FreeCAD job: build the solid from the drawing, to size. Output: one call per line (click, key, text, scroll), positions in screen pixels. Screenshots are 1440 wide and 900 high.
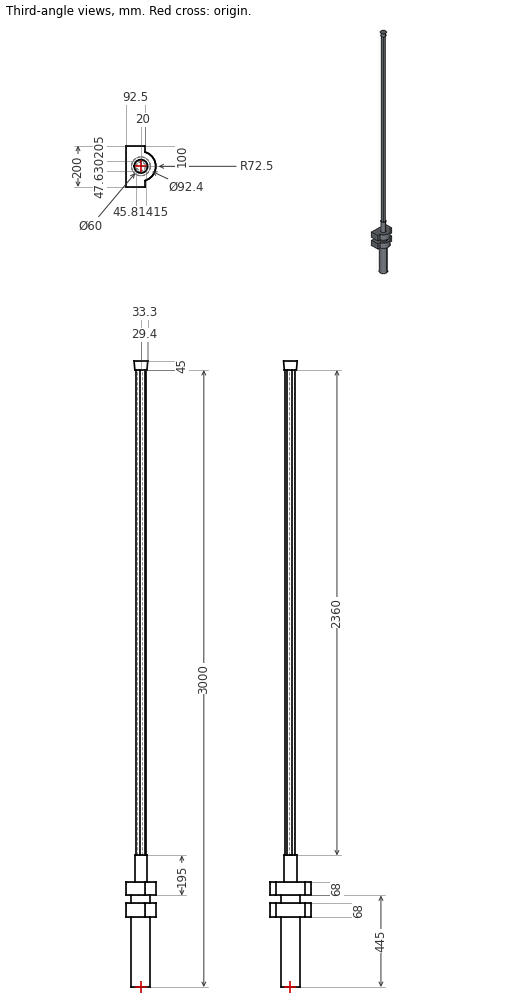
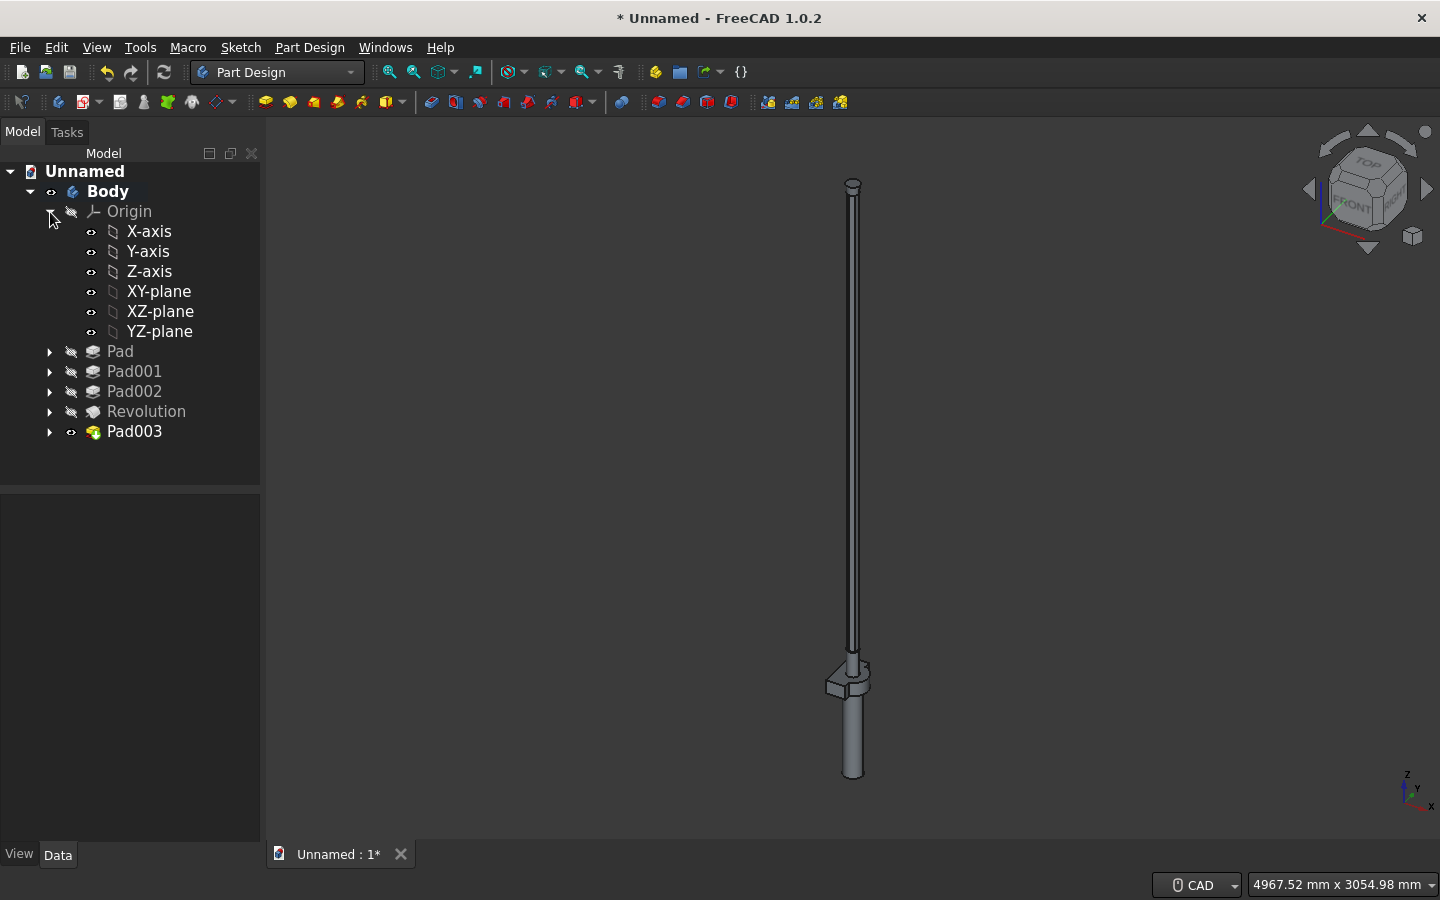
click(136, 292)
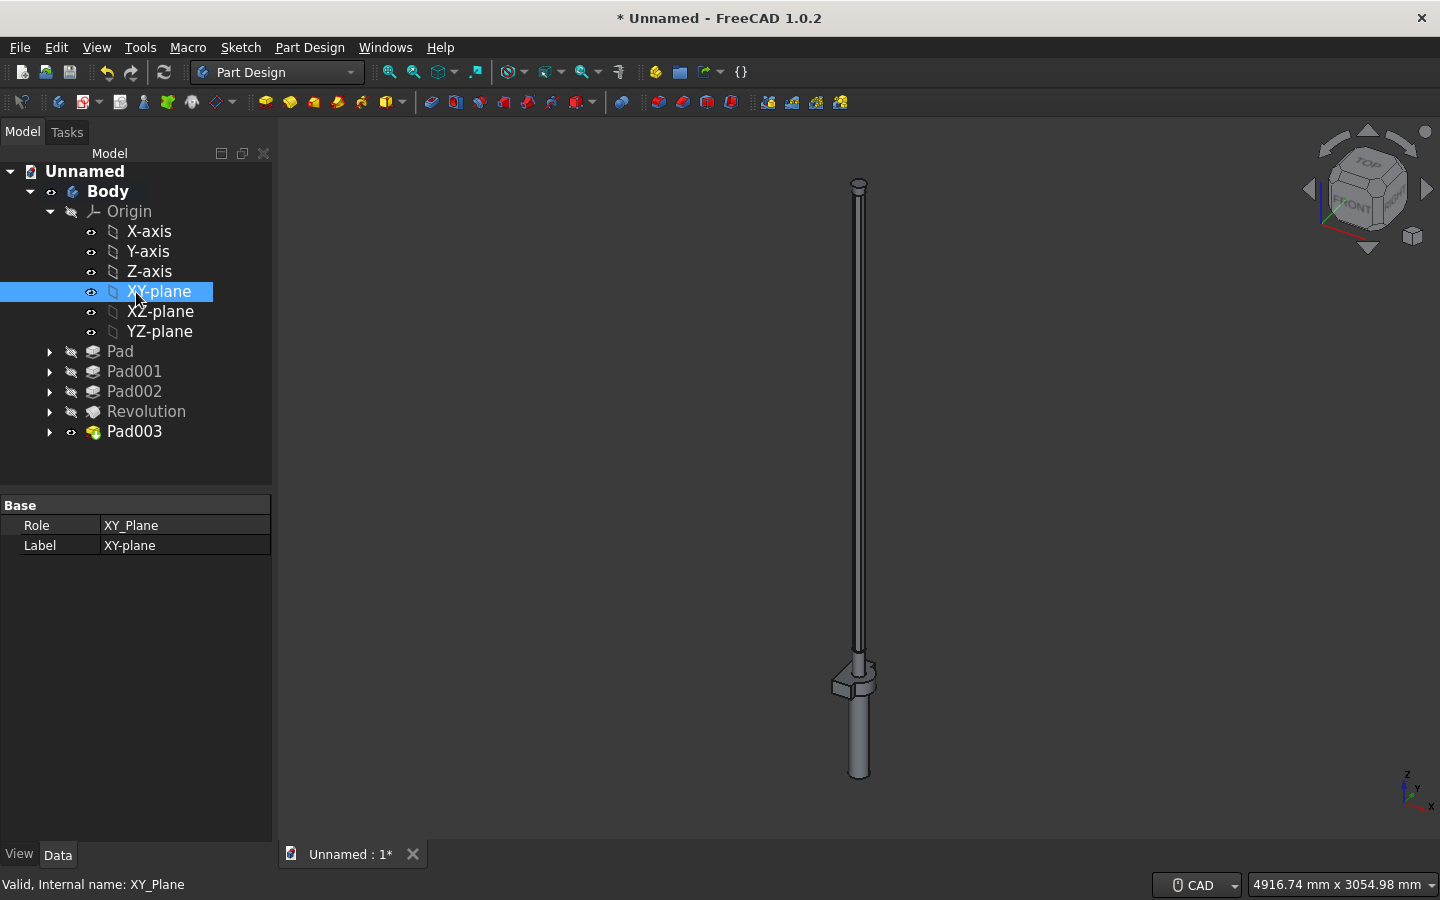
click(216, 102)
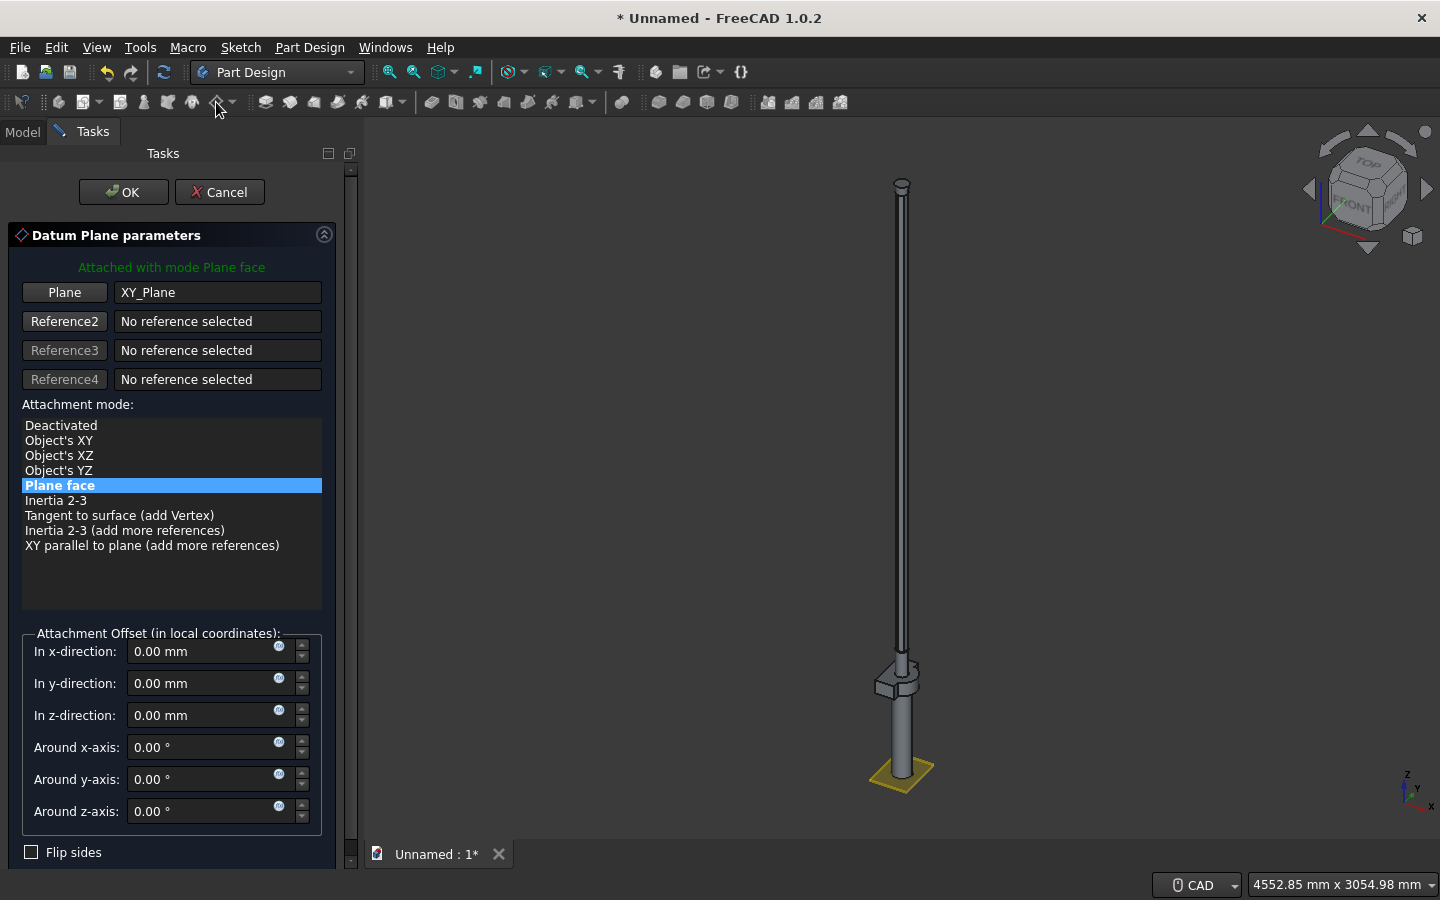
triple_click(210, 715)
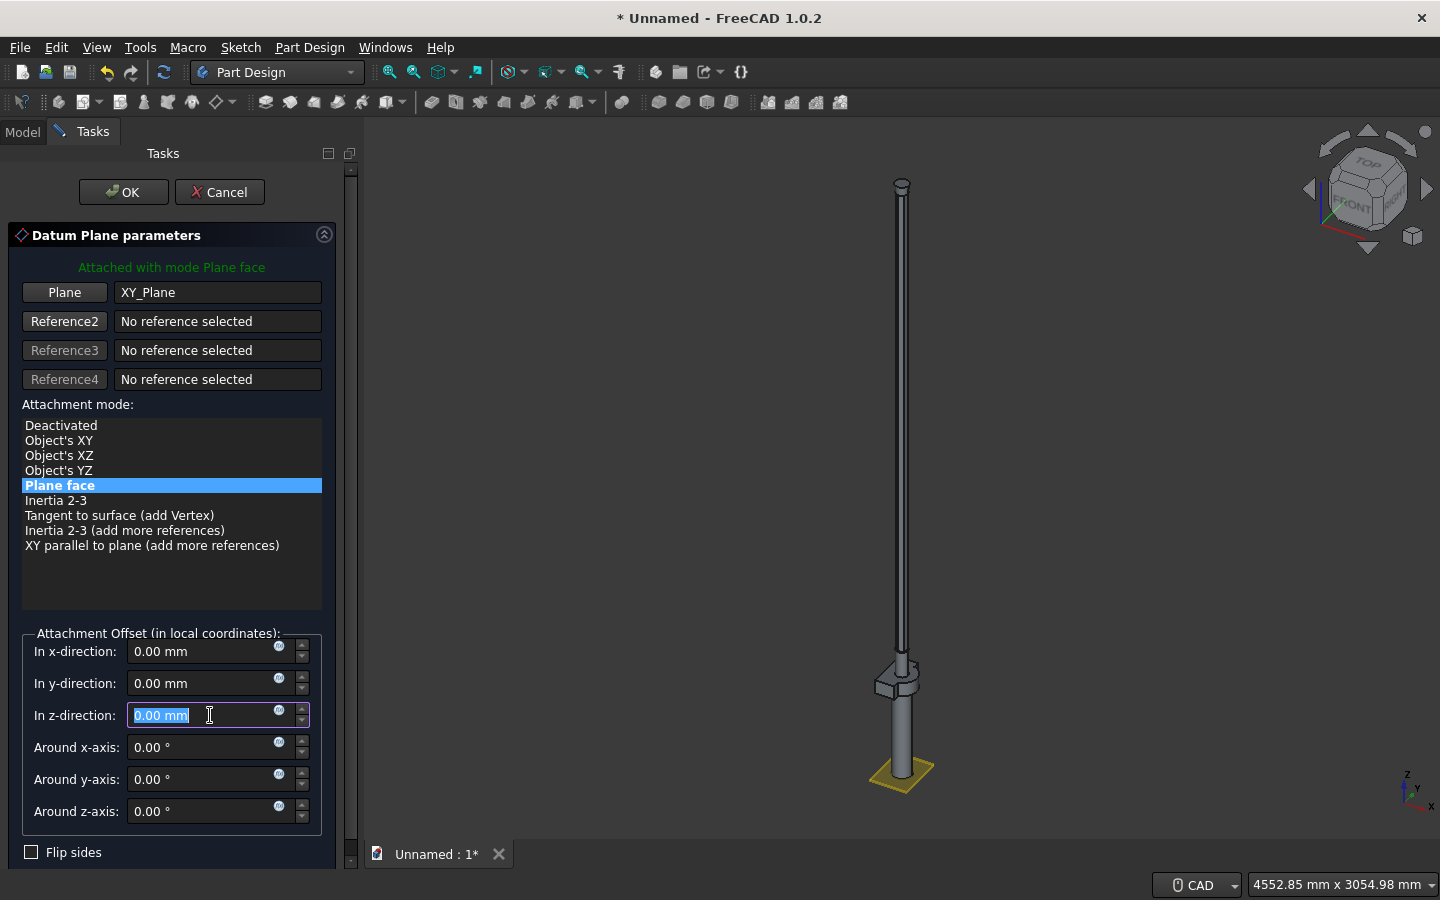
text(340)
key(Tab)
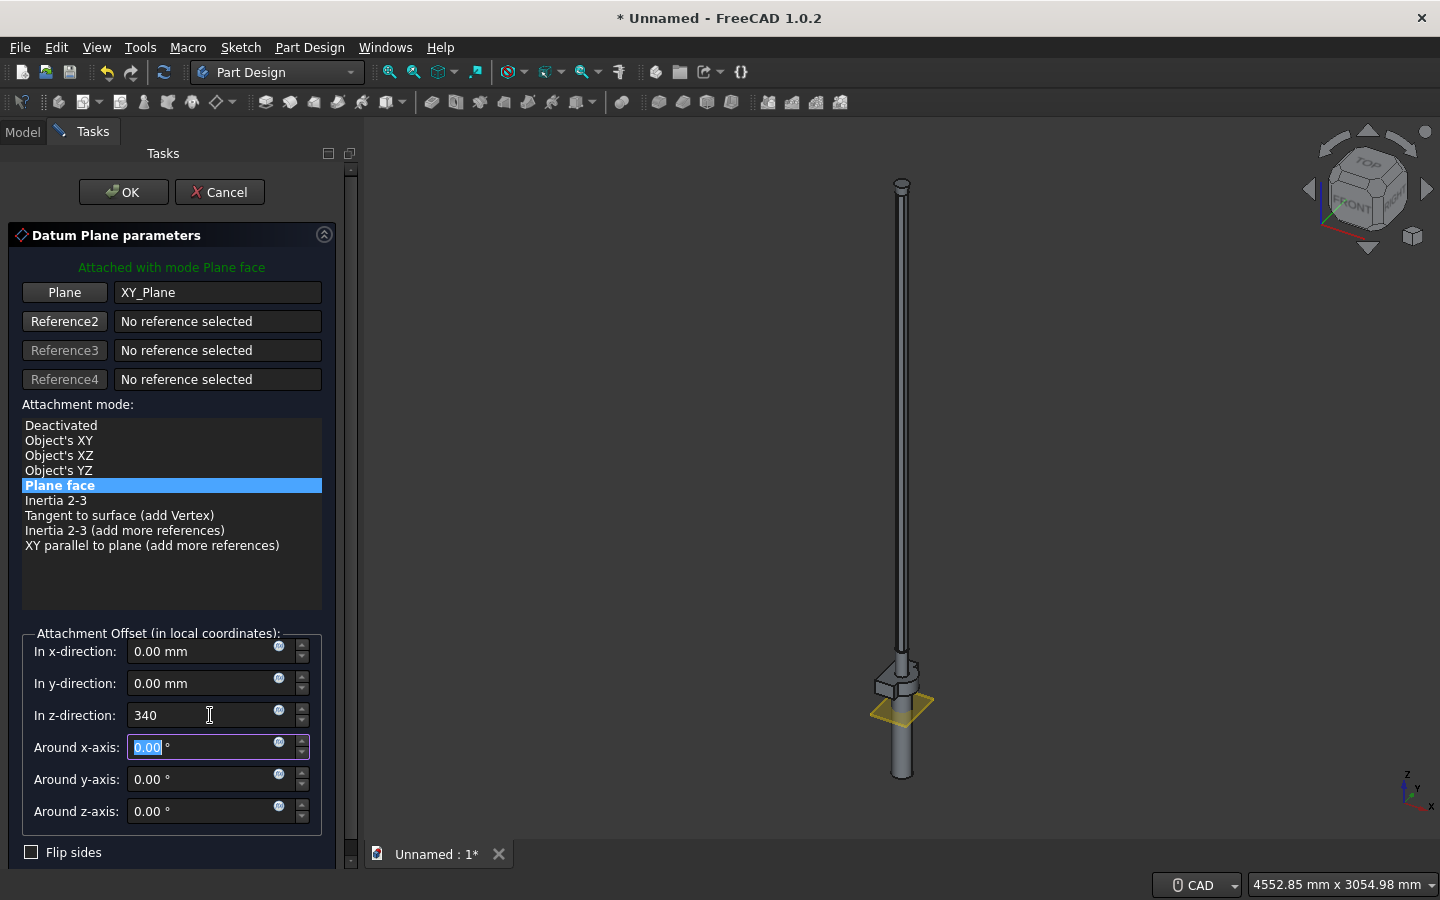
click(124, 192)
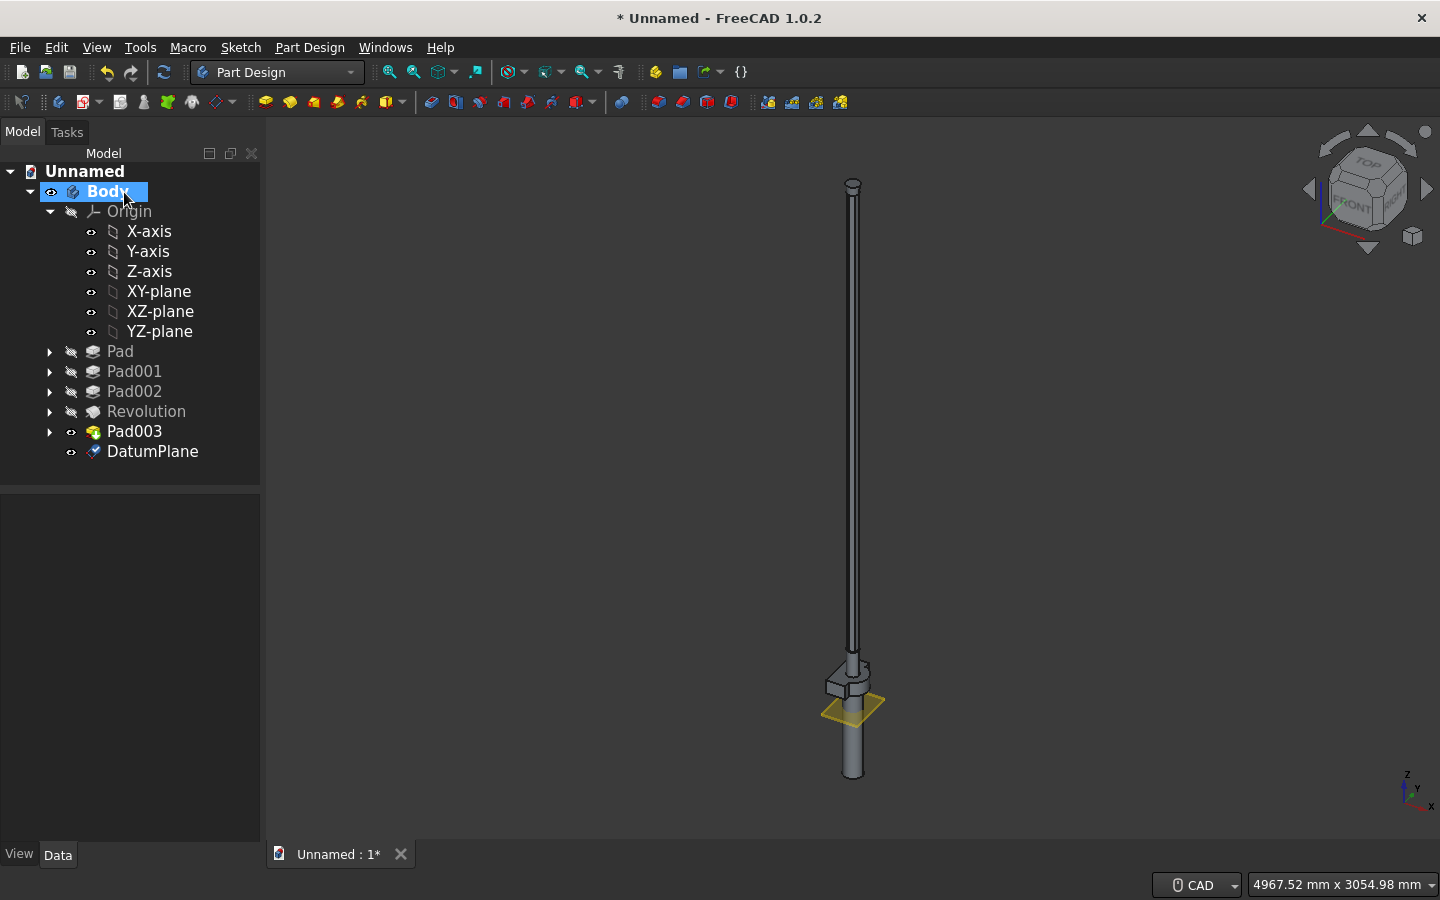
click(116, 452)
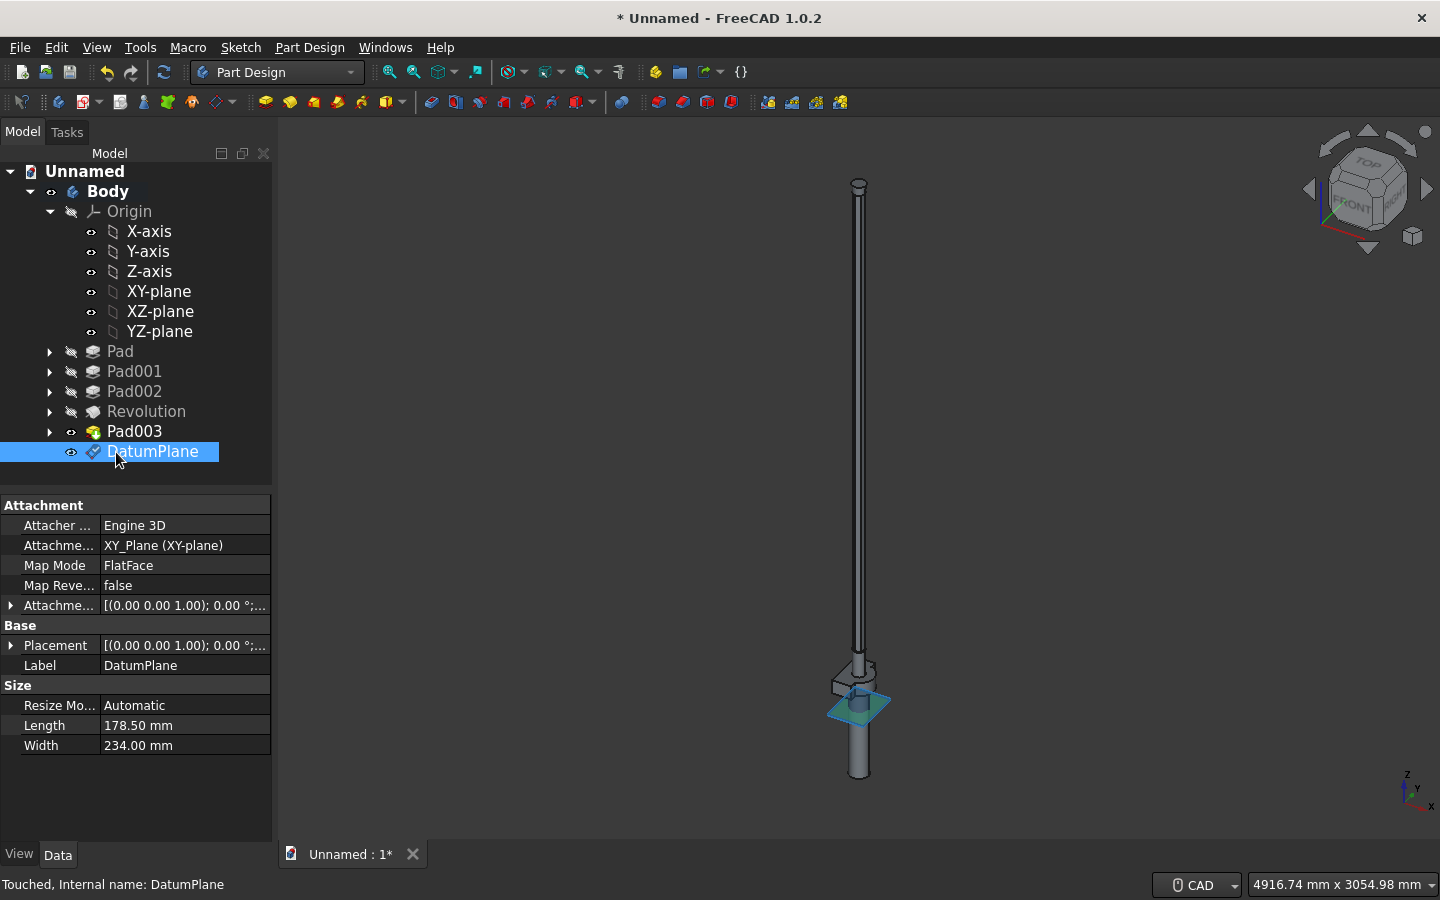
click(84, 102)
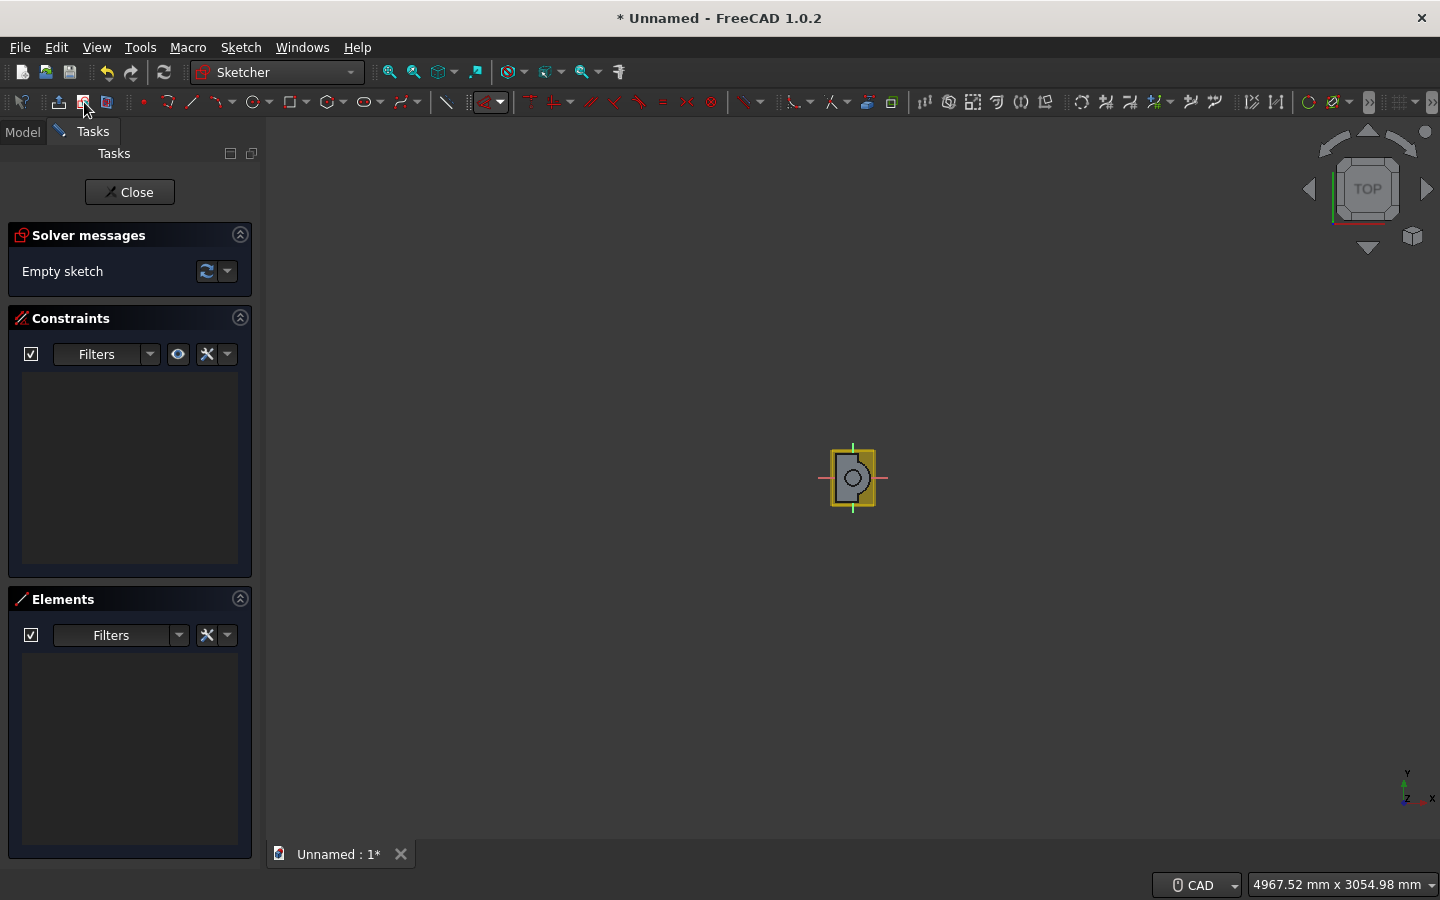
key(q)
key(s)